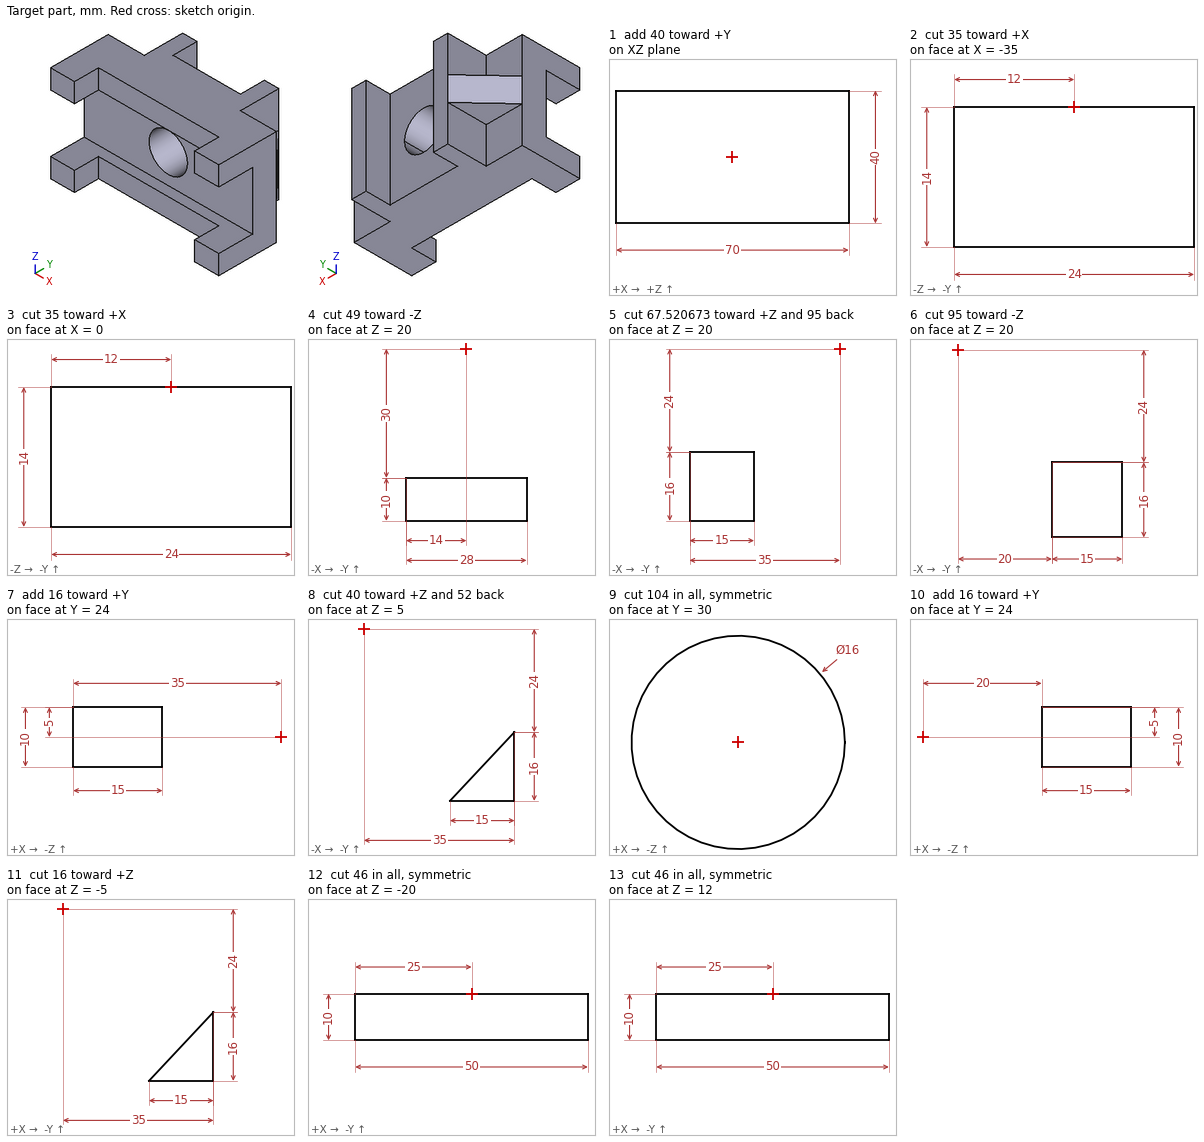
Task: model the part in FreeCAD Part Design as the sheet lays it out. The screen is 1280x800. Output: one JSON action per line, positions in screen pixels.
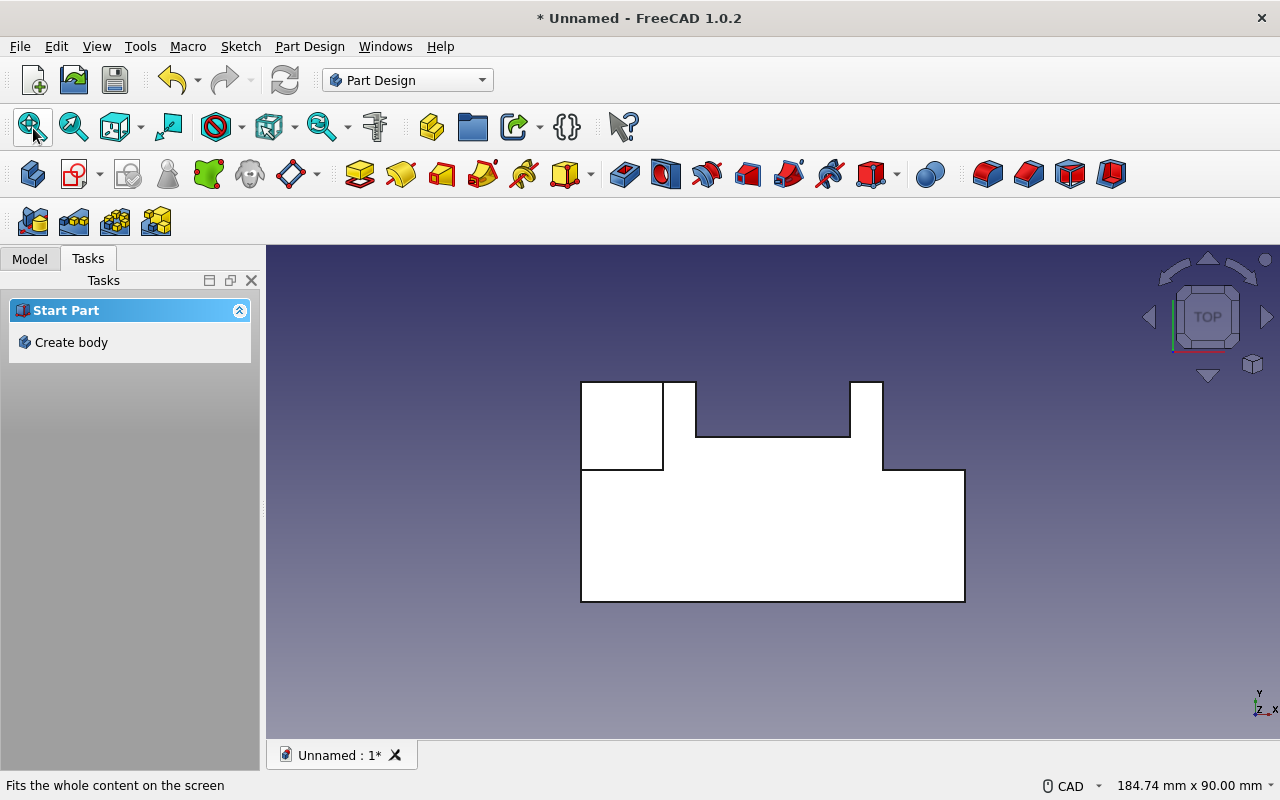
{"action": "left_click", "coordinate": [622, 425]}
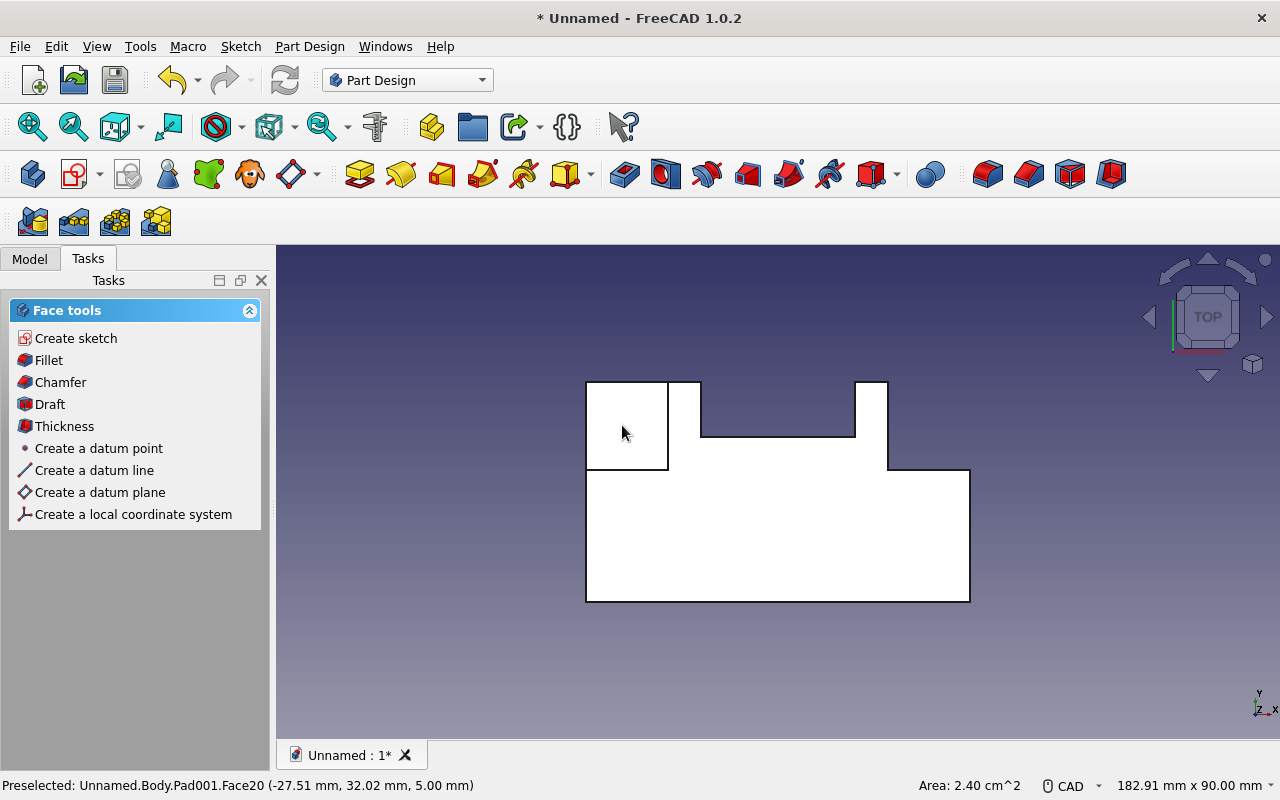
{"action": "left_click", "coordinate": [74, 174]}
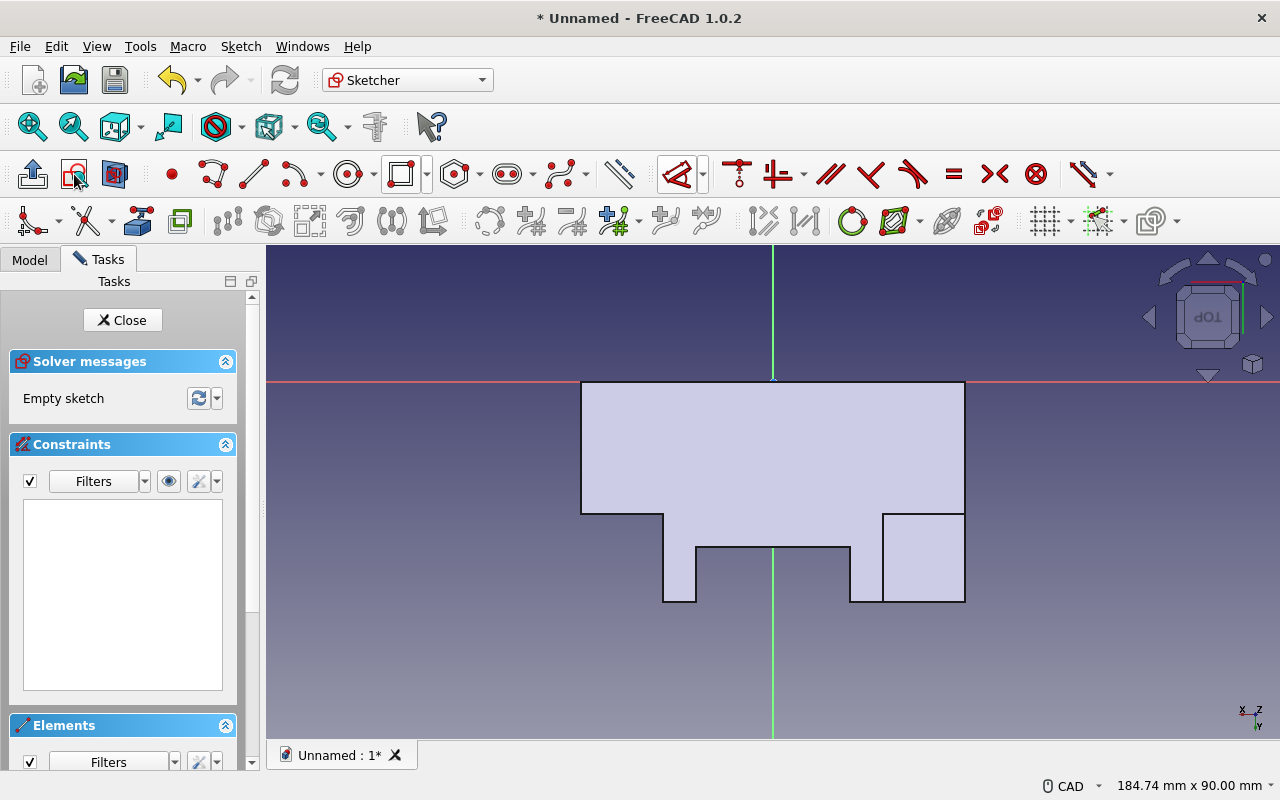
{"action": "left_click", "coordinate": [115, 174]}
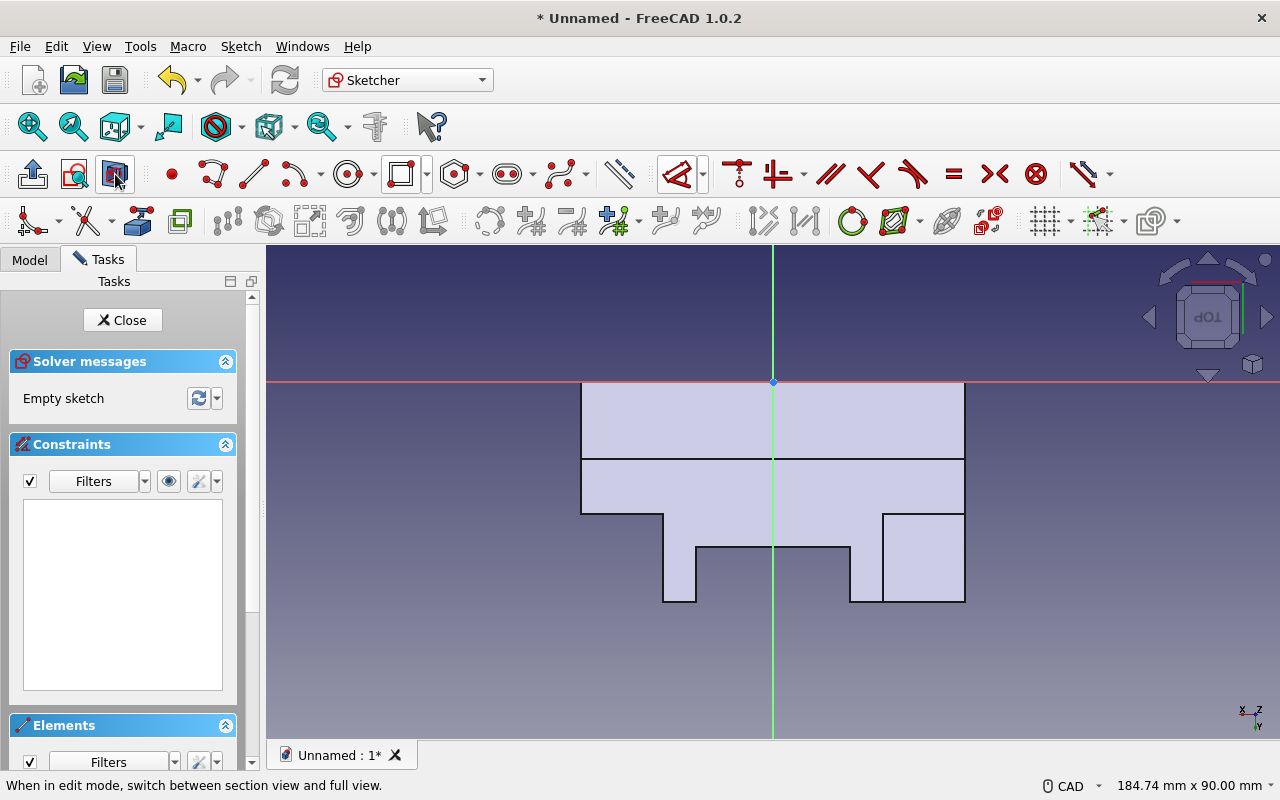
{"action": "scroll", "coordinate": [1019, 586], "scroll_direction": "up", "scroll_amount": 6}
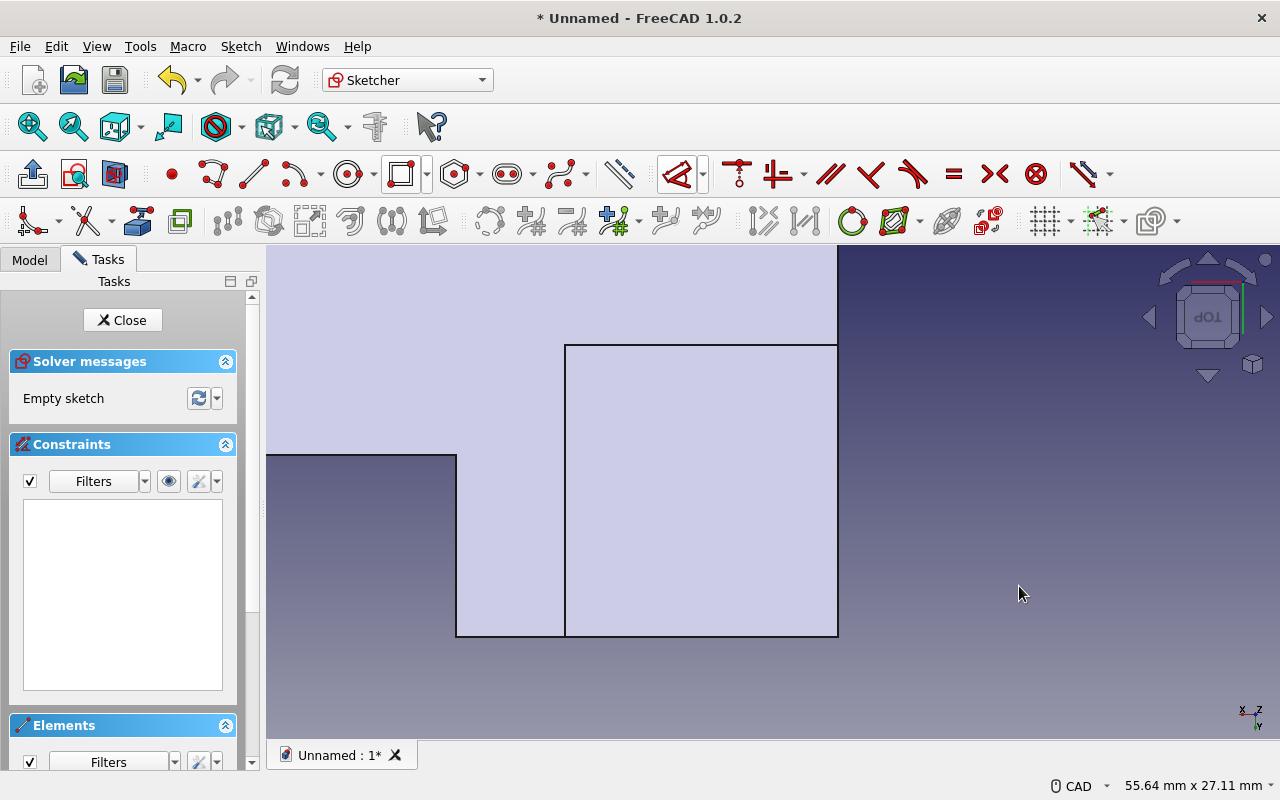
{"action": "key", "text": "g m"}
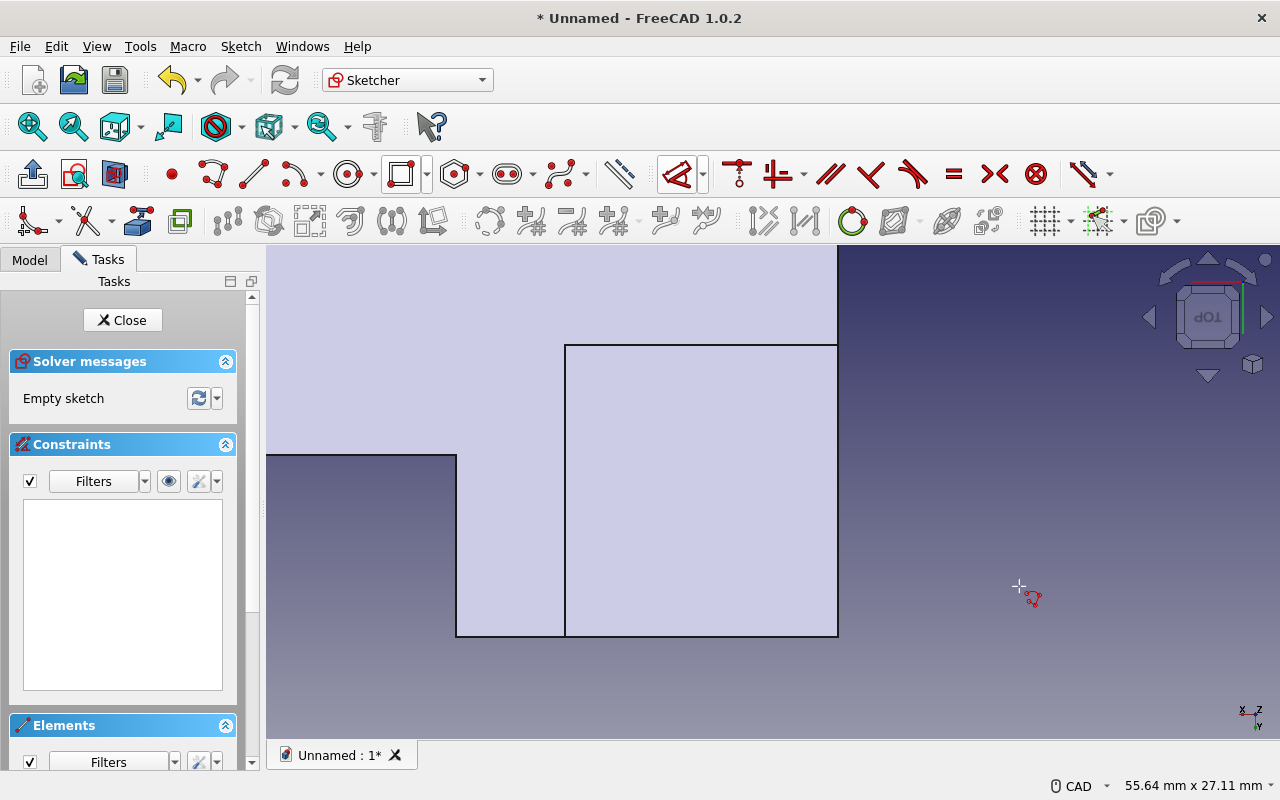
{"action": "left_click", "coordinate": [838, 345]}
{"action": "left_click", "coordinate": [565, 637]}
{"action": "left_click", "coordinate": [838, 637]}
{"action": "left_click", "coordinate": [838, 346]}
{"action": "key", "text": "Escape"}
{"action": "key", "text": "Escape"}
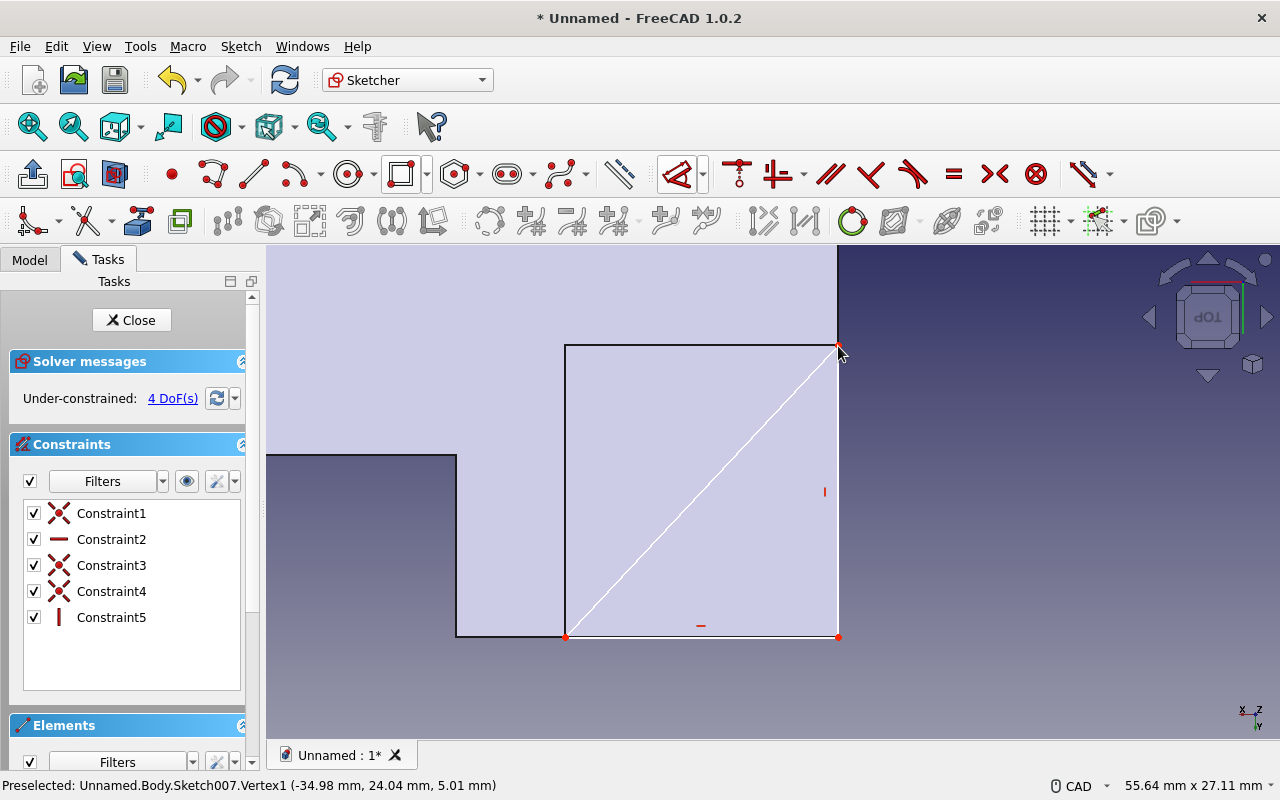
{"action": "left_click", "coordinate": [647, 638]}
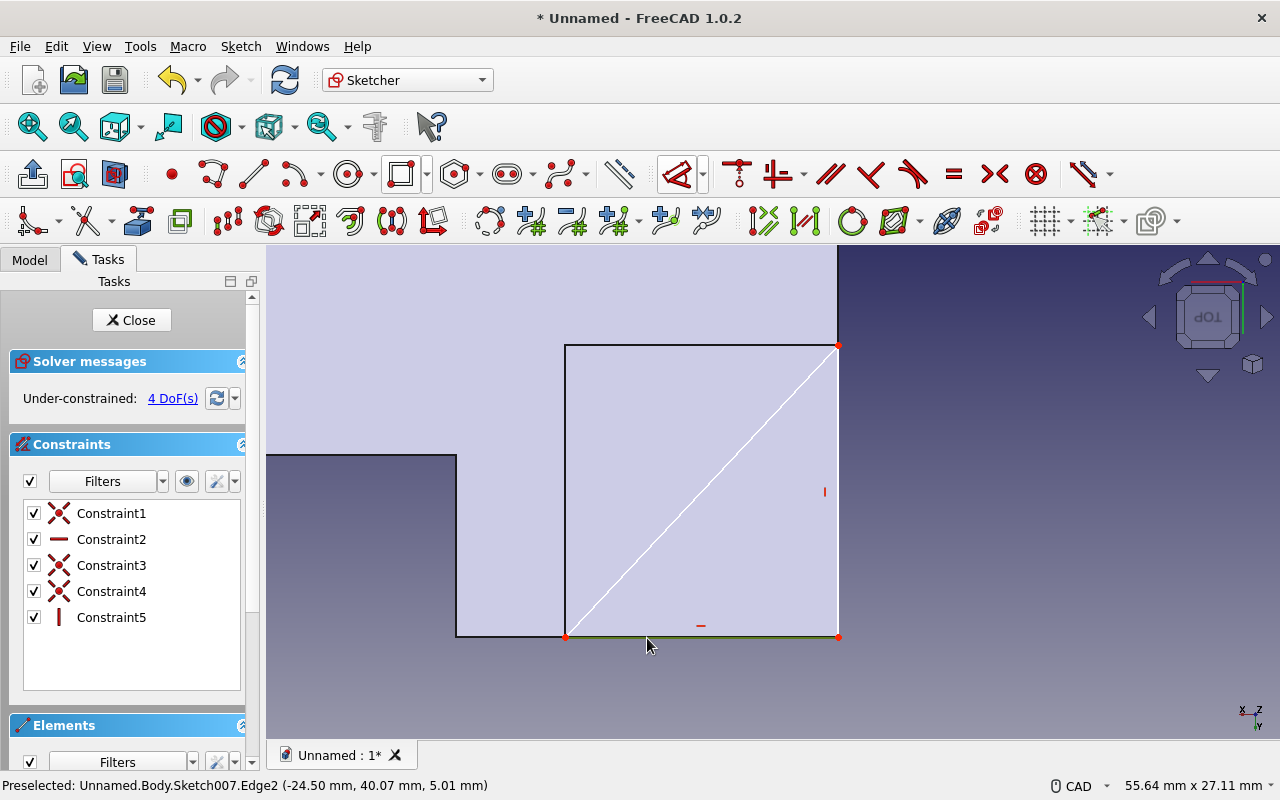
{"action": "key", "text": "l"}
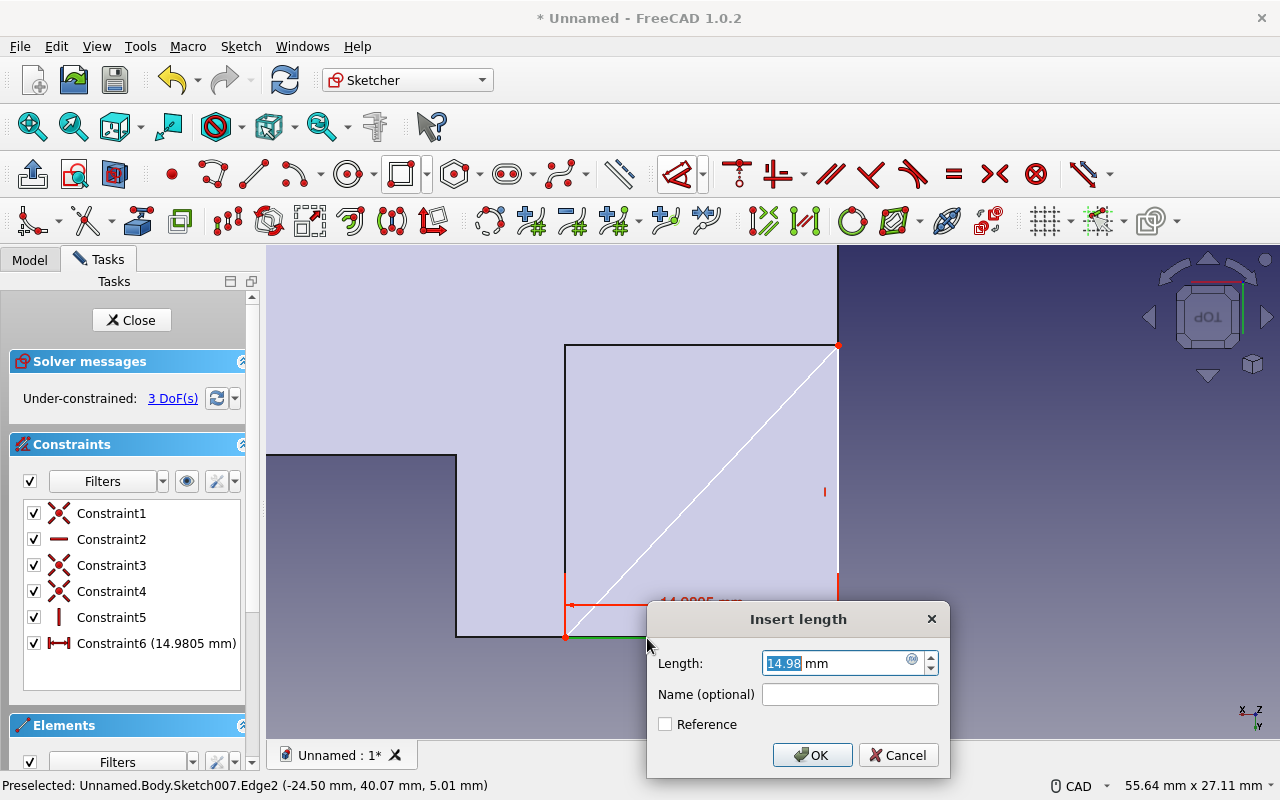
{"action": "type", "text": "15"}
{"action": "key", "text": "Return"}